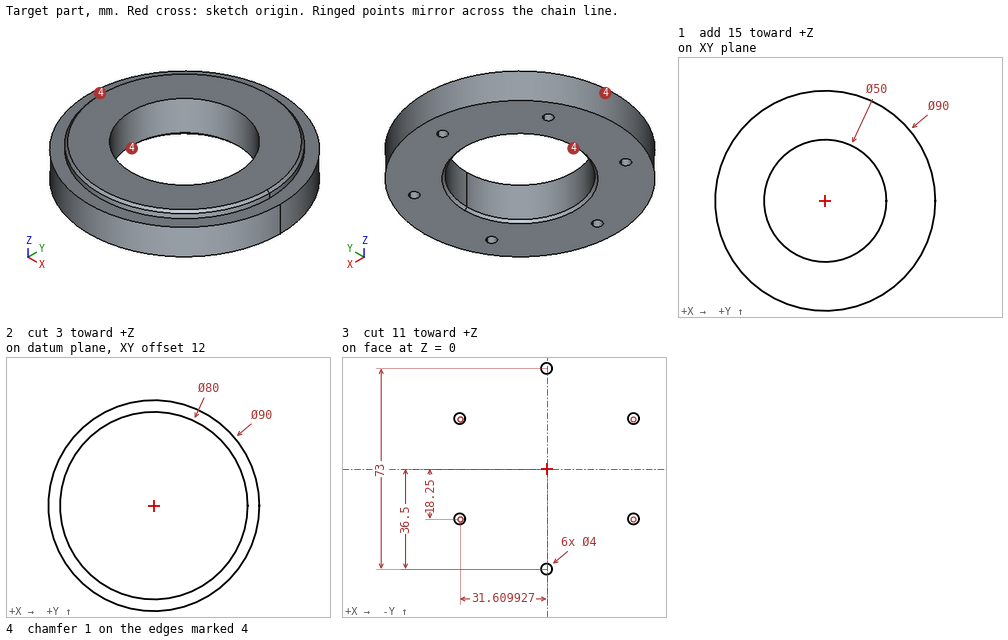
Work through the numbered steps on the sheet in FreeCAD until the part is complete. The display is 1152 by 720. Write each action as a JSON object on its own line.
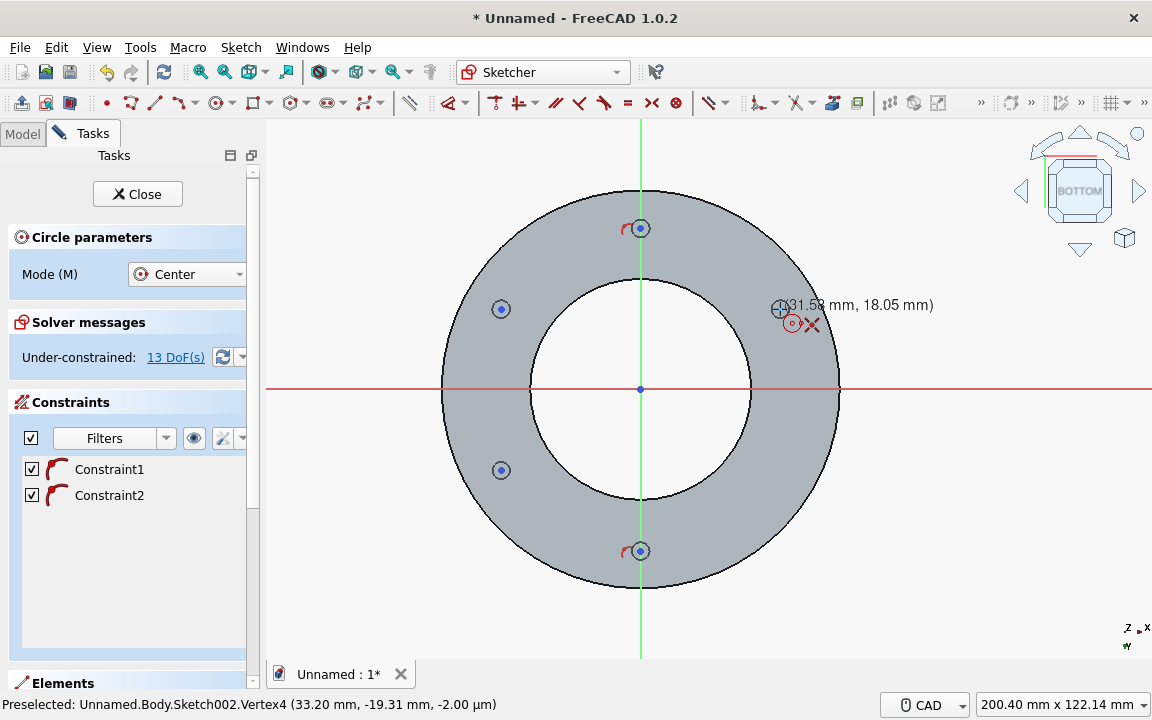
{"action": "scroll", "coordinate": [780, 470], "scroll_direction": "up", "scroll_amount": 5}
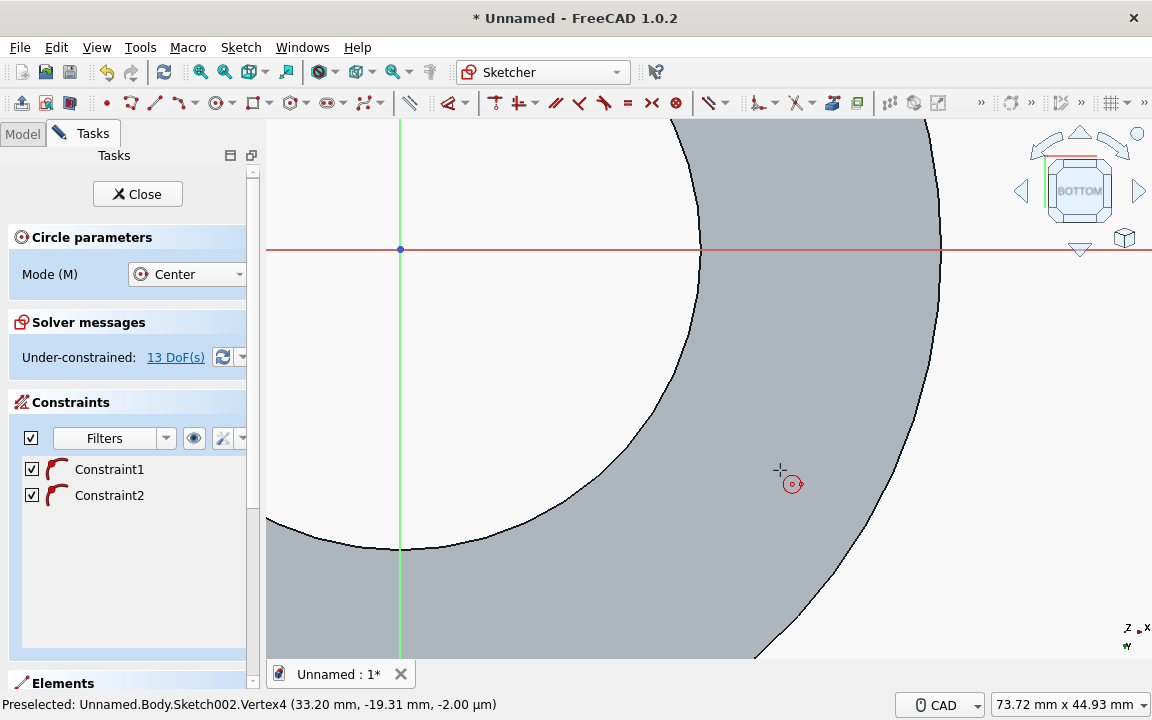
{"action": "left_click", "coordinate": [780, 469]}
{"action": "left_click", "coordinate": [797, 452]}
{"action": "key", "text": "Escape"}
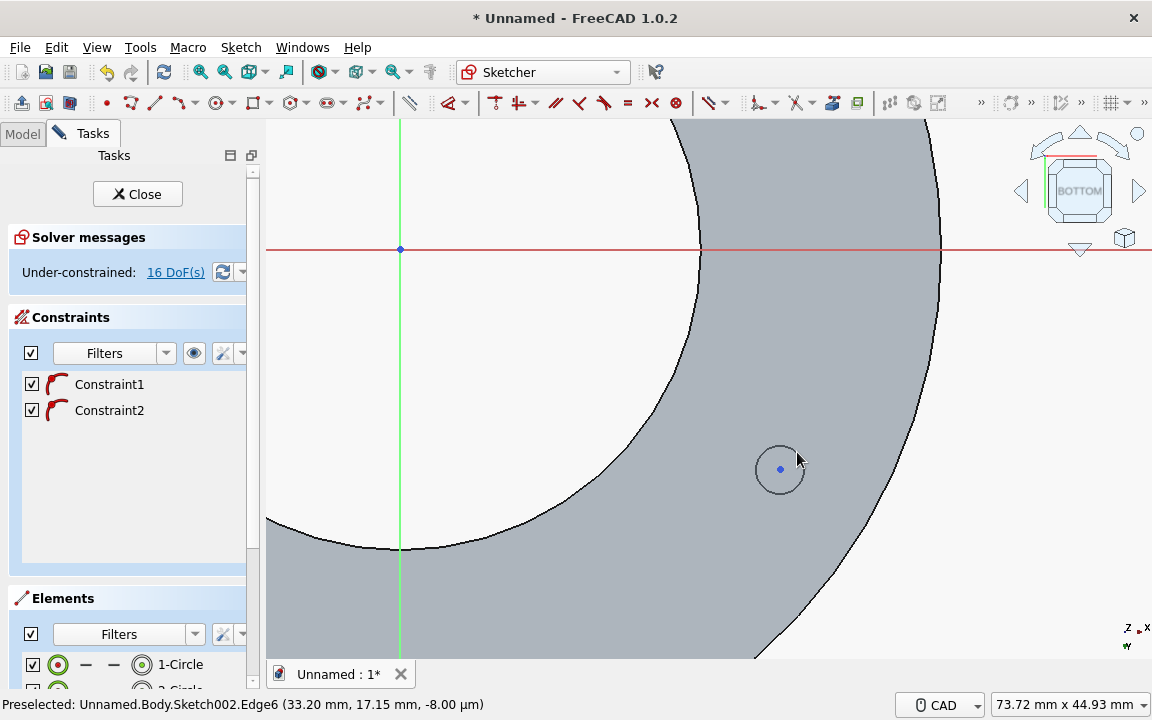
{"action": "scroll", "coordinate": [780, 470], "scroll_direction": "down", "scroll_amount": 5}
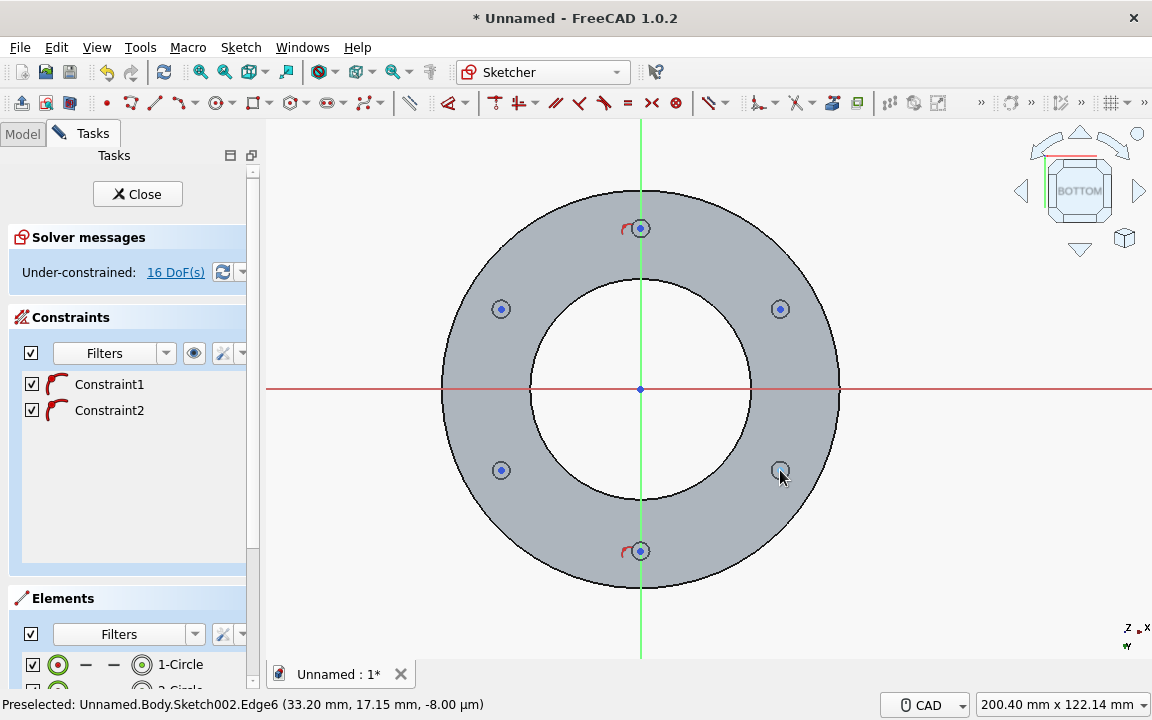
{"action": "scroll", "coordinate": [647, 545], "scroll_direction": "up", "scroll_amount": 5}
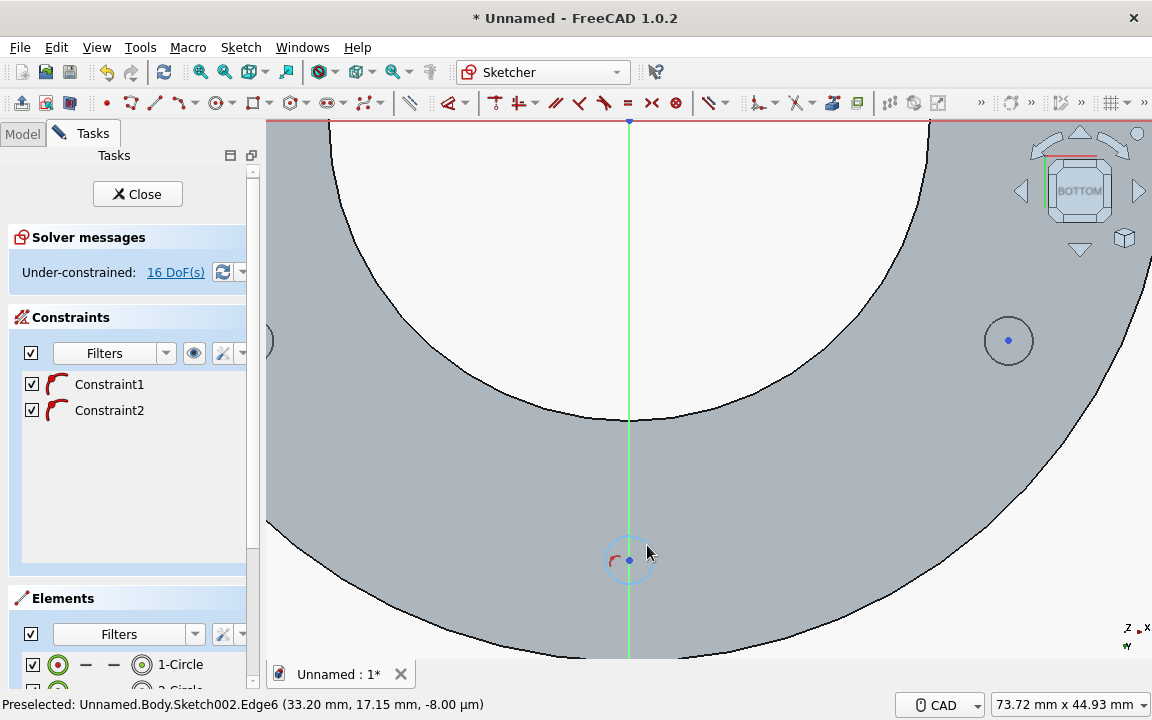
{"action": "left_click", "coordinate": [646, 543]}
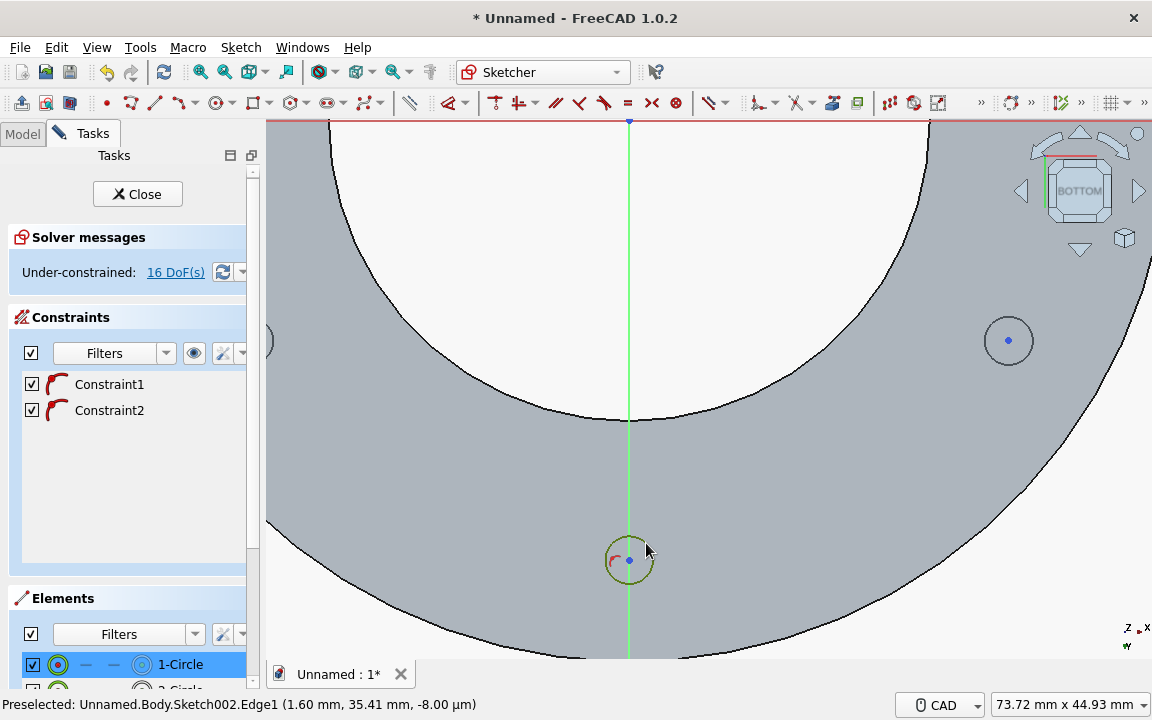
{"action": "scroll", "coordinate": [647, 545], "scroll_direction": "down", "scroll_amount": 5}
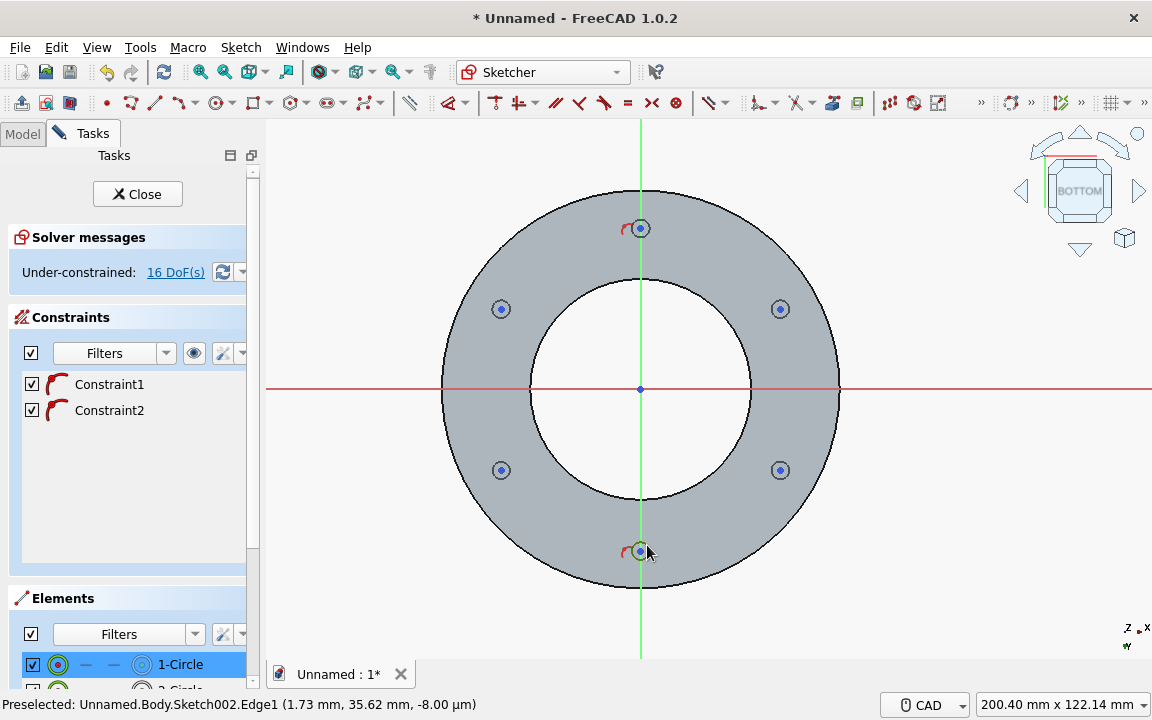
{"action": "scroll", "coordinate": [507, 464], "scroll_direction": "up", "scroll_amount": 3}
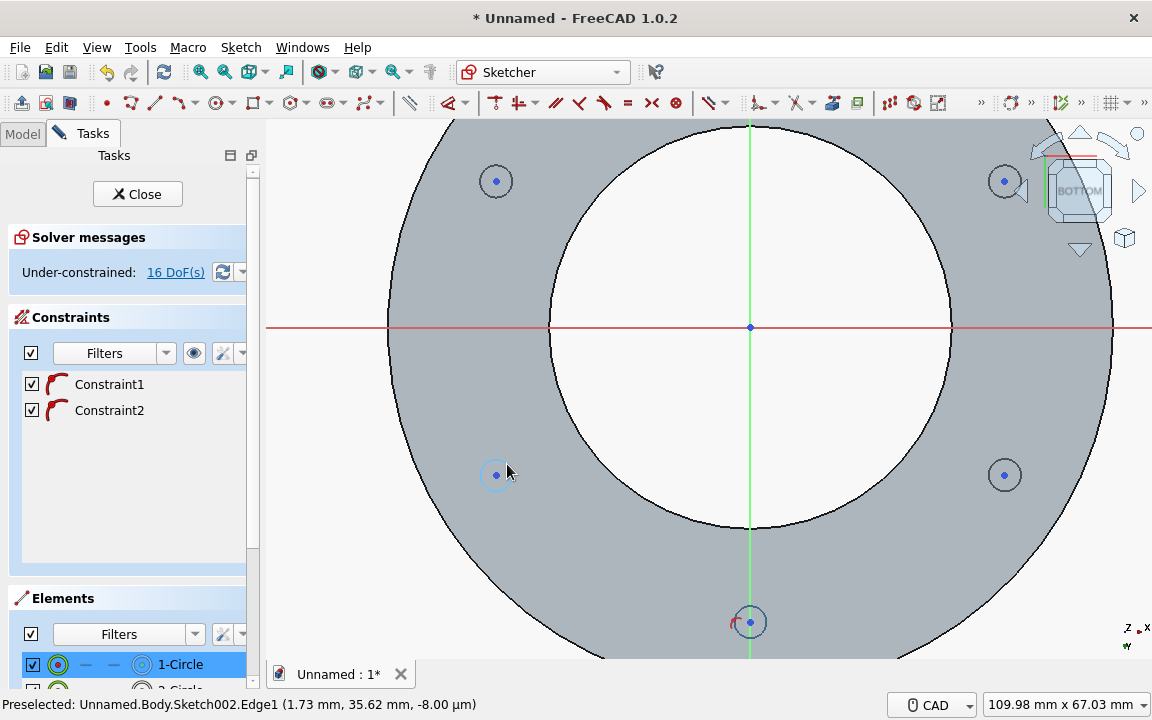
{"action": "left_click", "coordinate": [507, 464]}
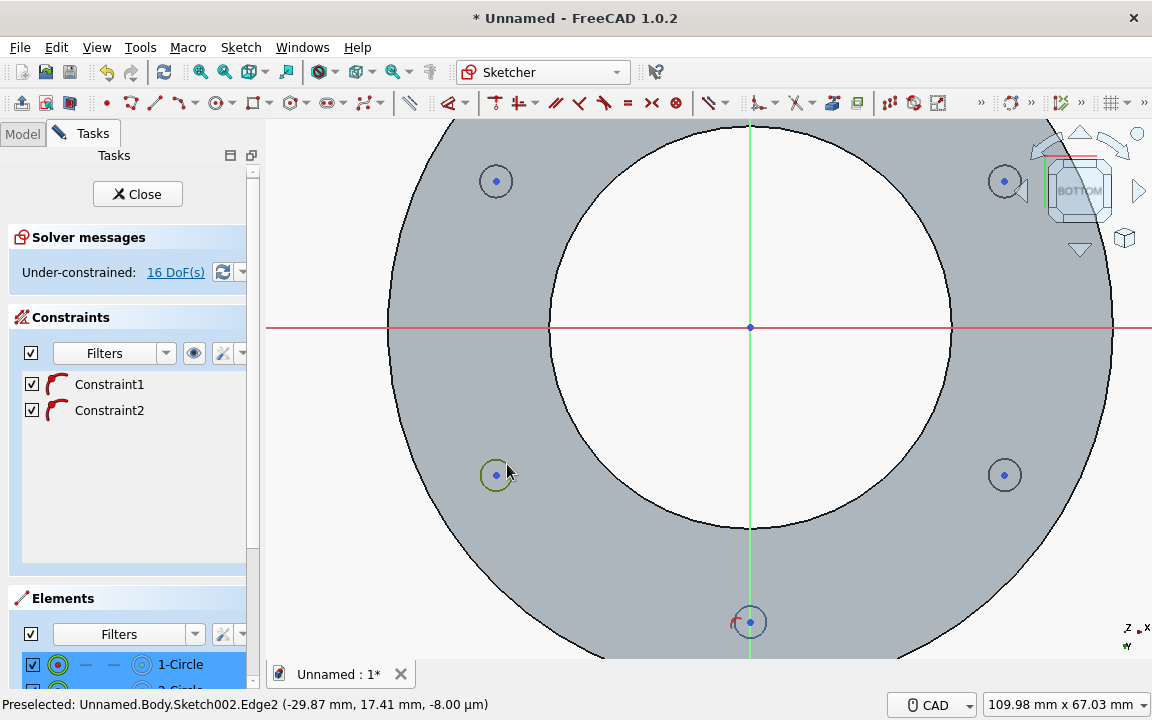
{"action": "left_click", "coordinate": [508, 170]}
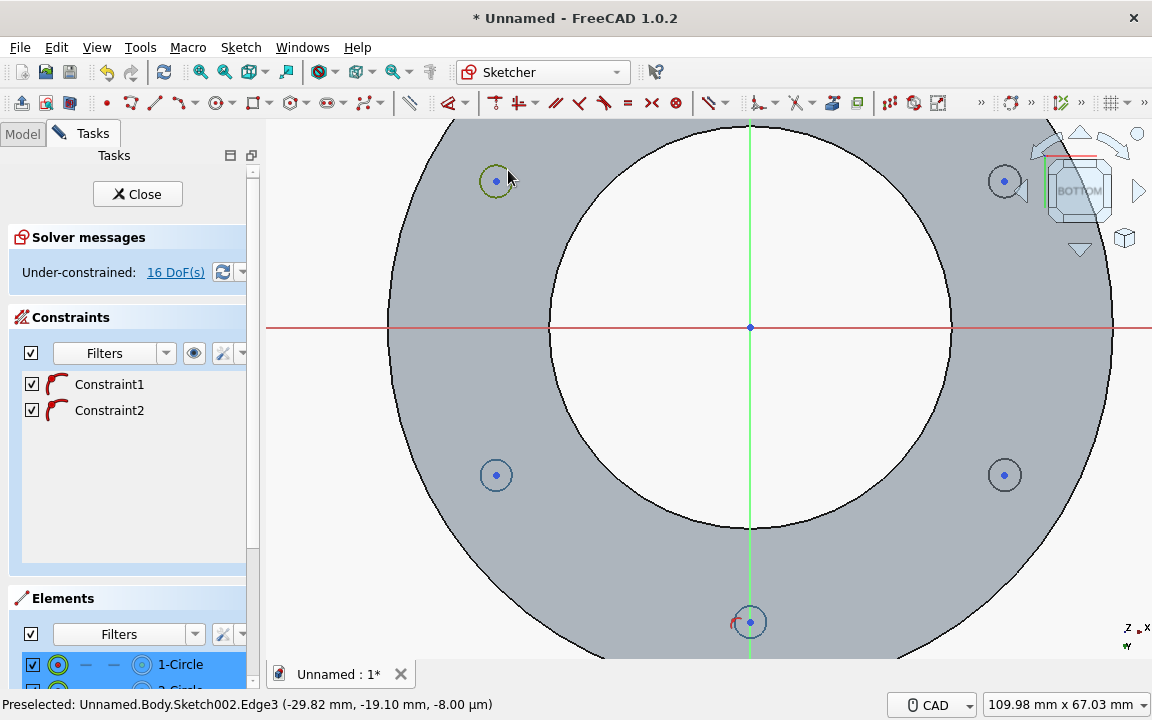
{"action": "scroll", "coordinate": [507, 464], "scroll_direction": "down", "scroll_amount": 3}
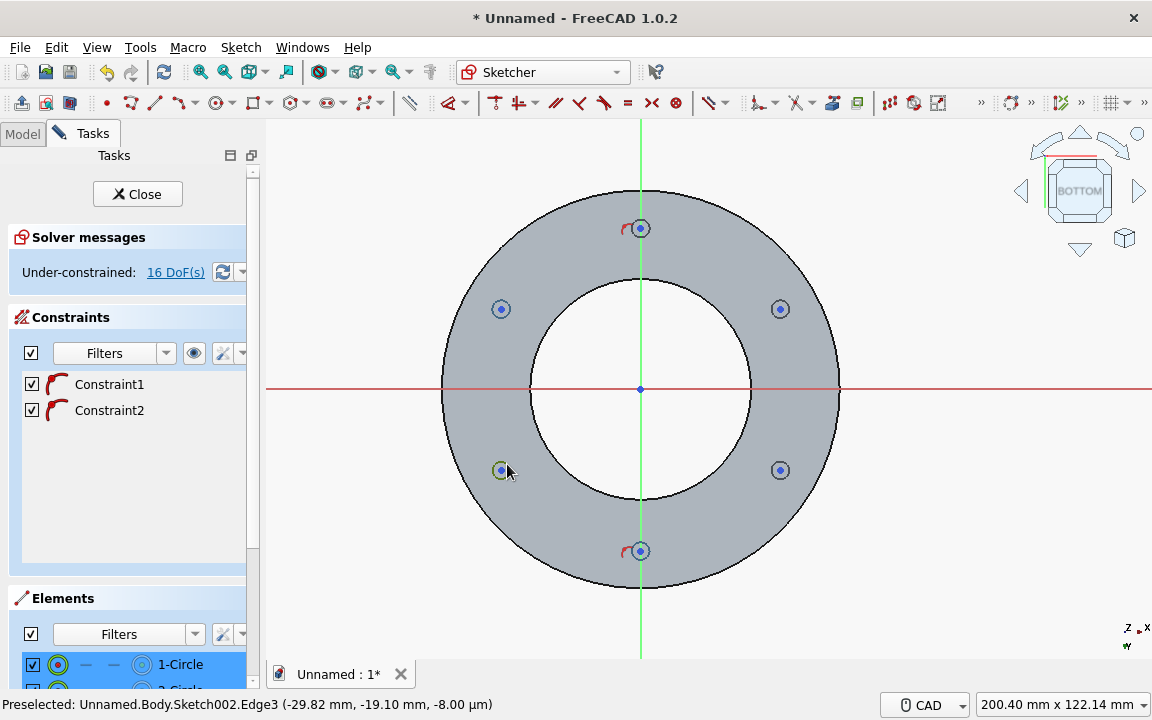
{"action": "scroll", "coordinate": [647, 222], "scroll_direction": "up", "scroll_amount": 4}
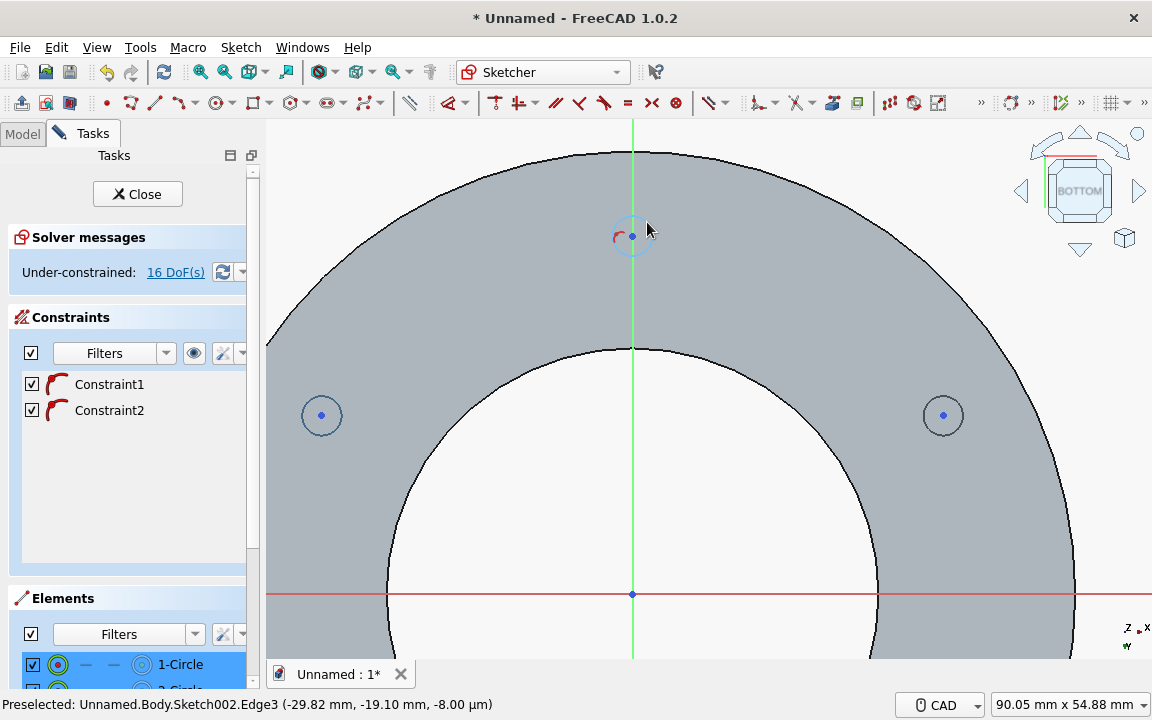
{"action": "left_click", "coordinate": [647, 222]}